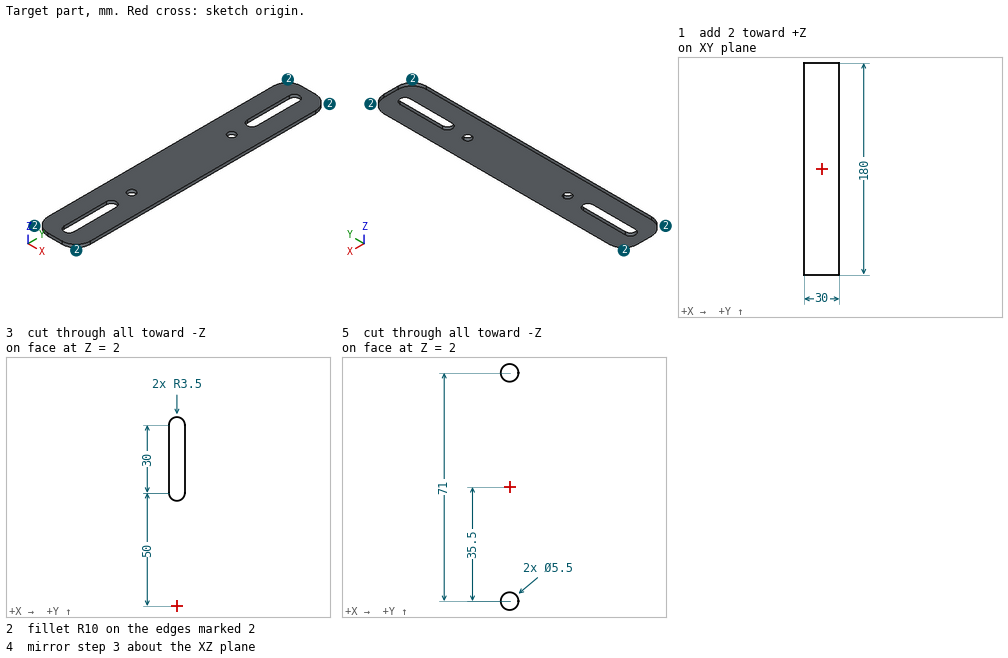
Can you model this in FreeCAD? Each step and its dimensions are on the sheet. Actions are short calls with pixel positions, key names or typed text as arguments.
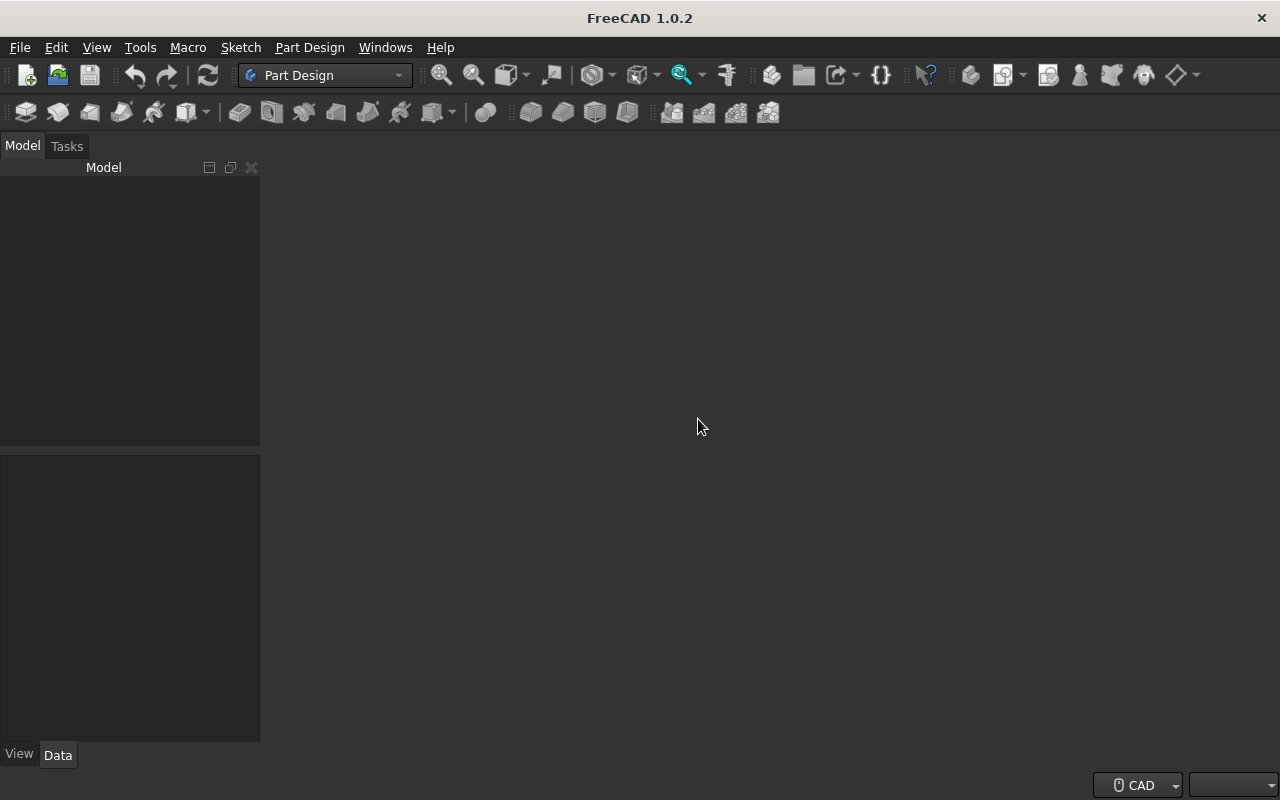
key(ctrl+n)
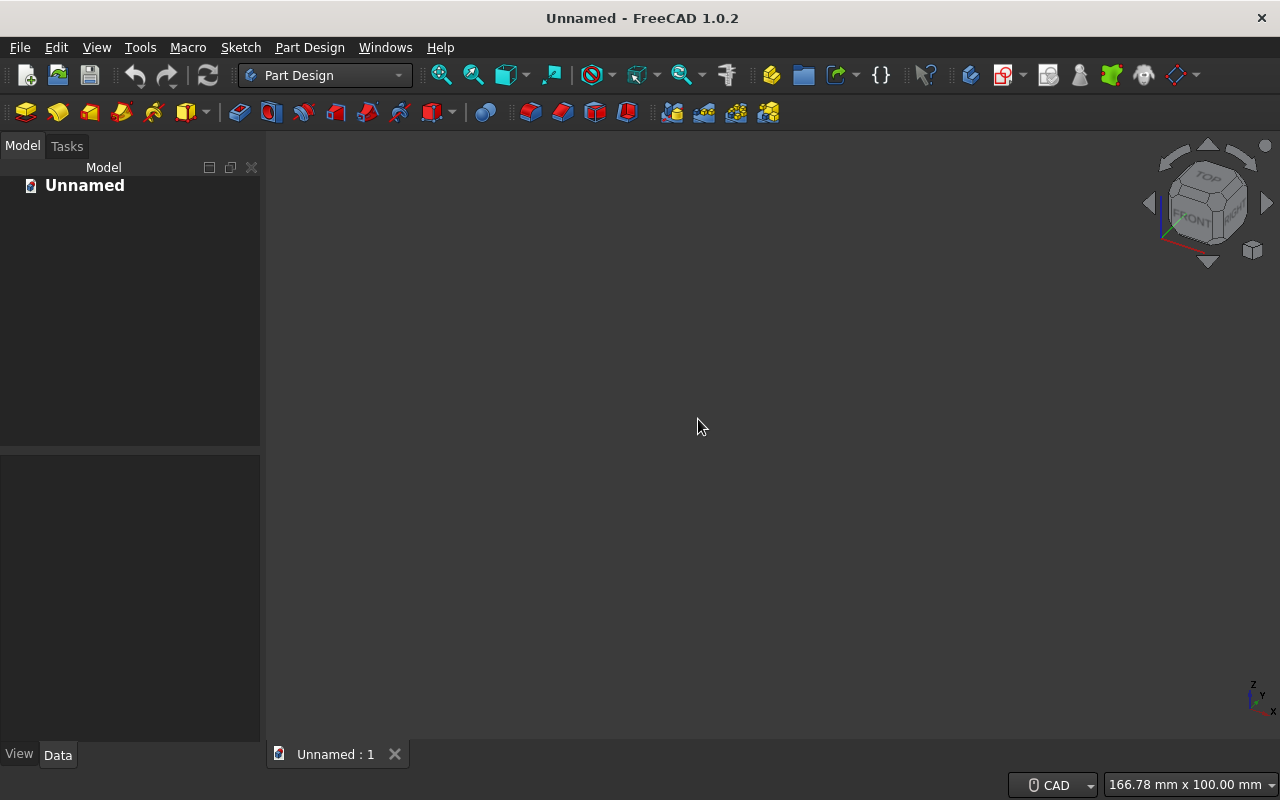
click(1004, 76)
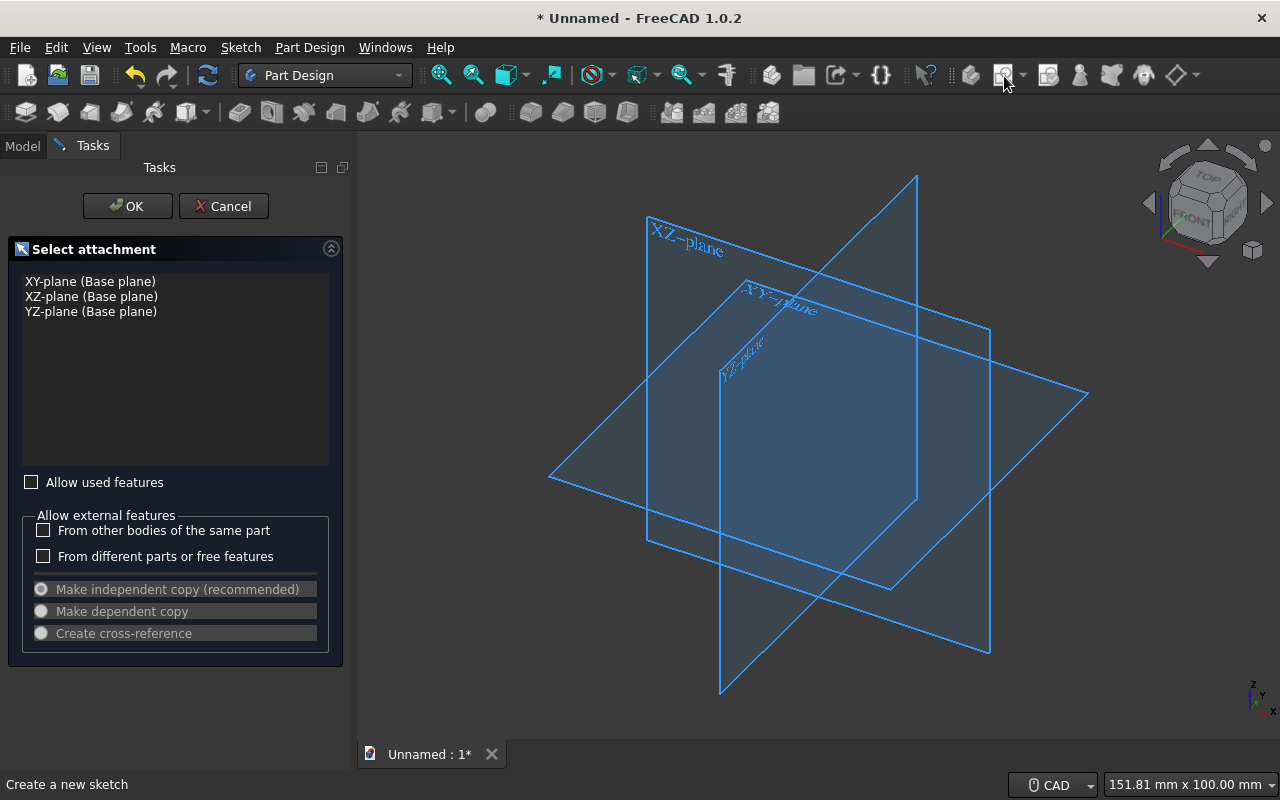
click(82, 282)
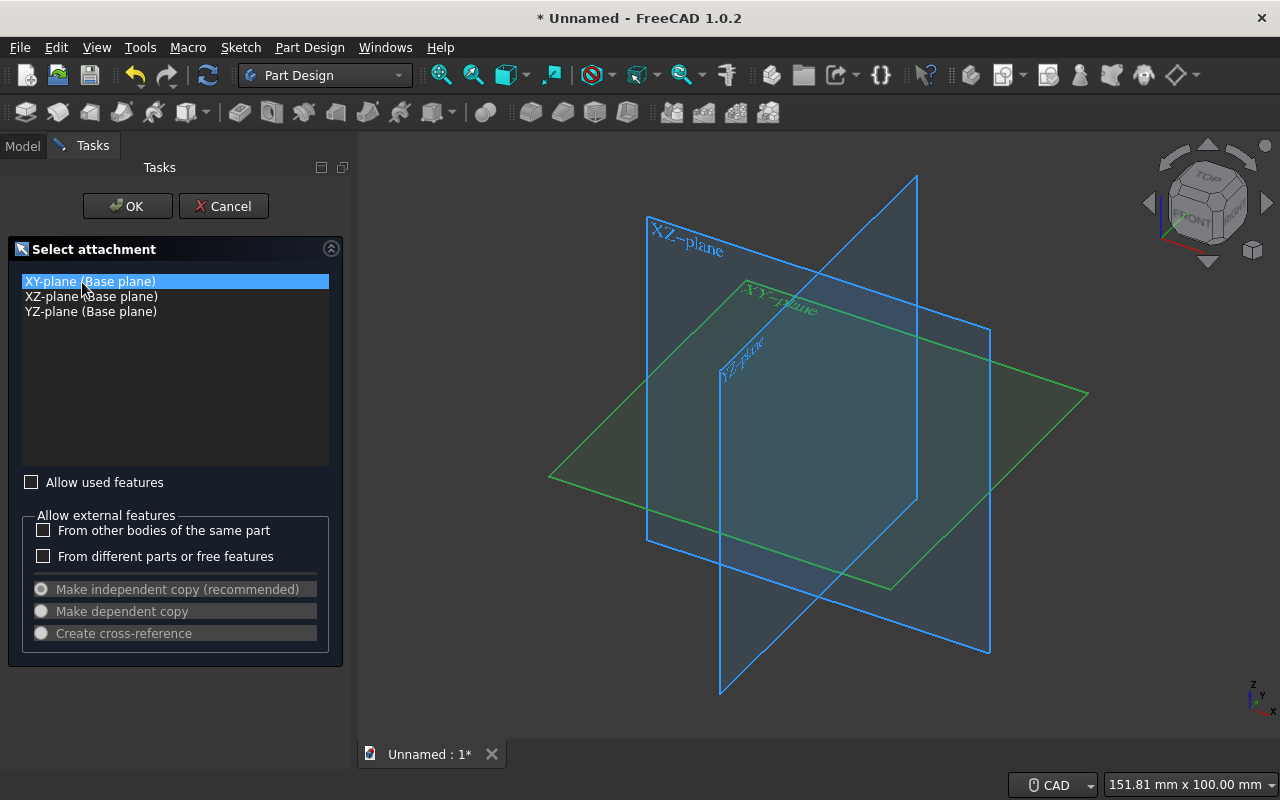
click(128, 206)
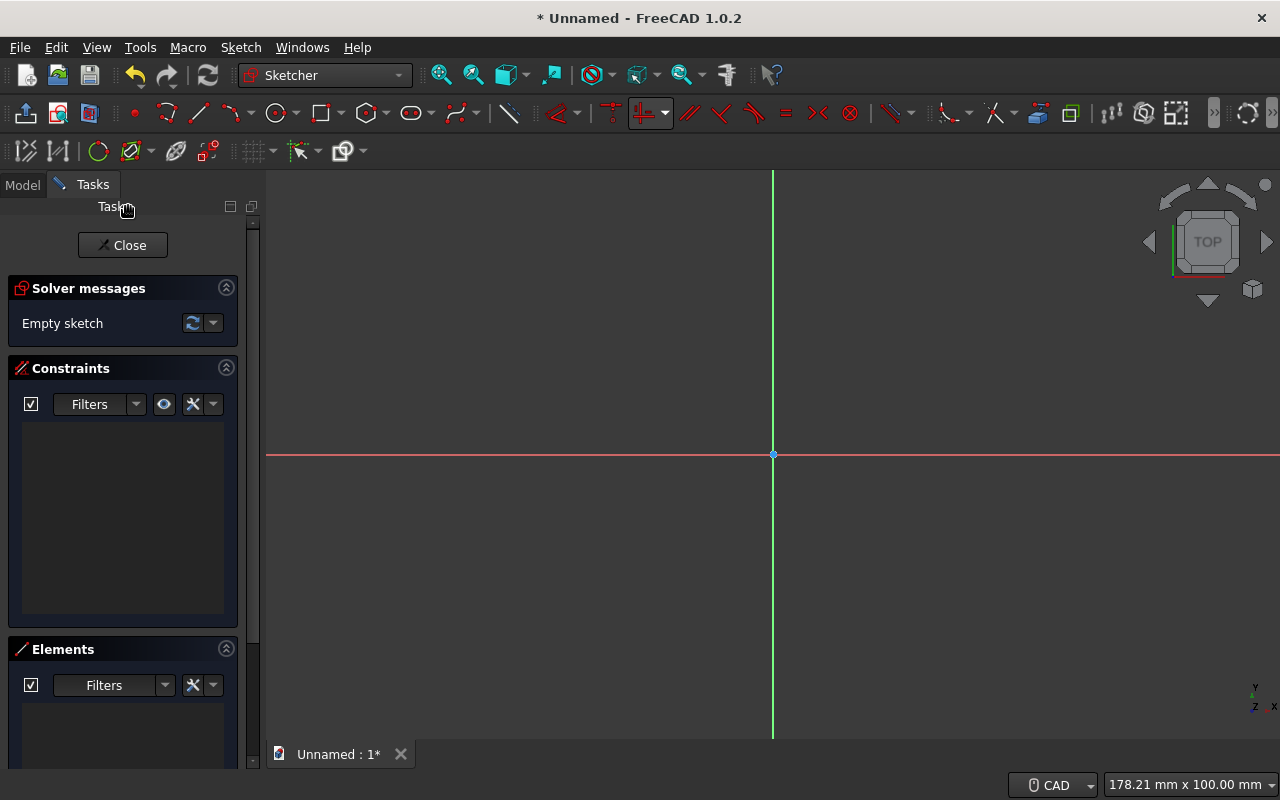
scroll(665, 454, down, 5)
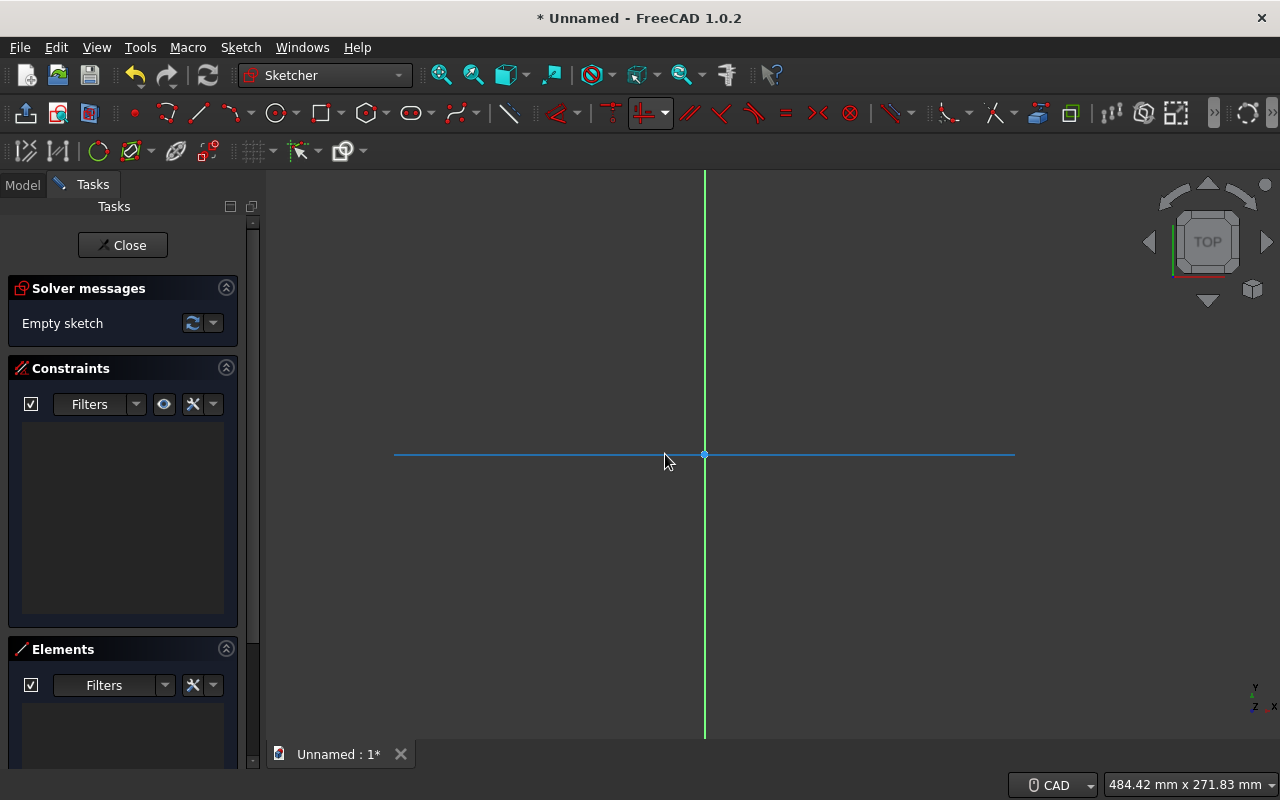
key(g)
key(v)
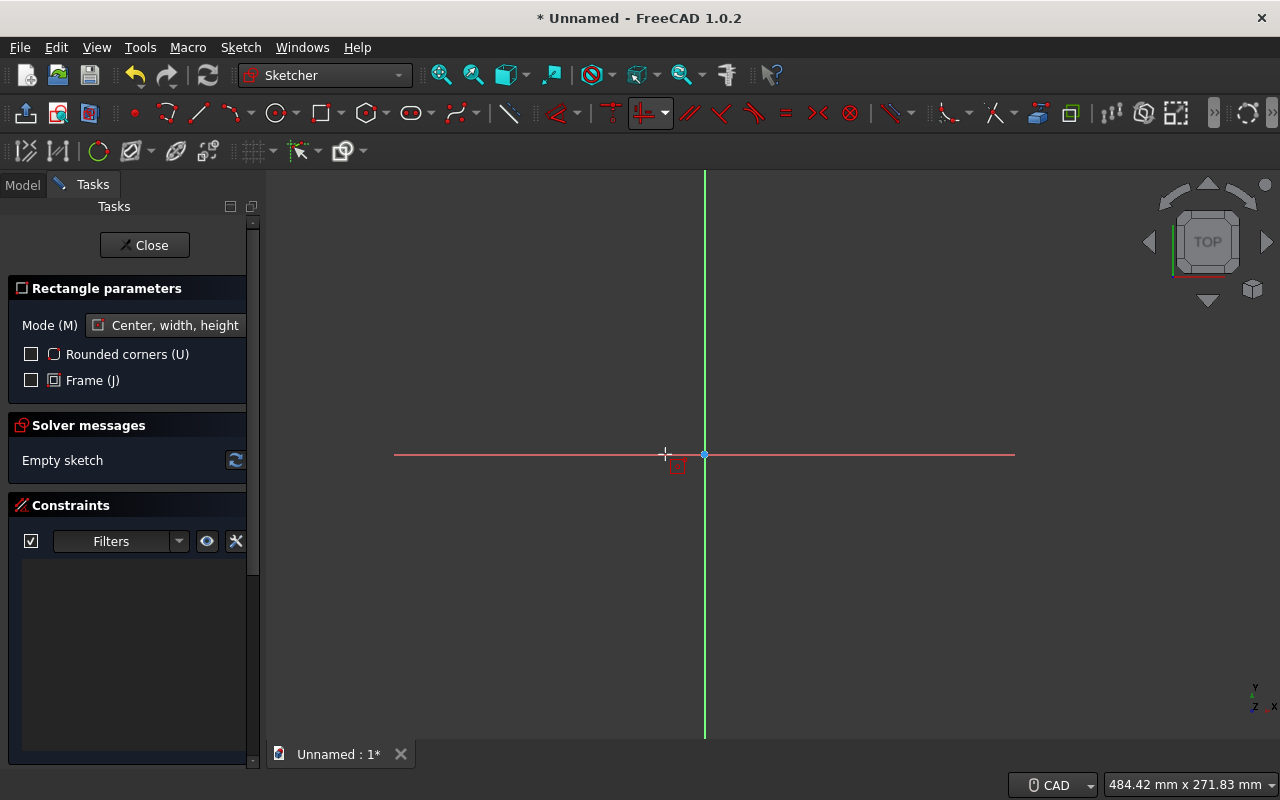
click(705, 454)
click(736, 266)
key(Escape)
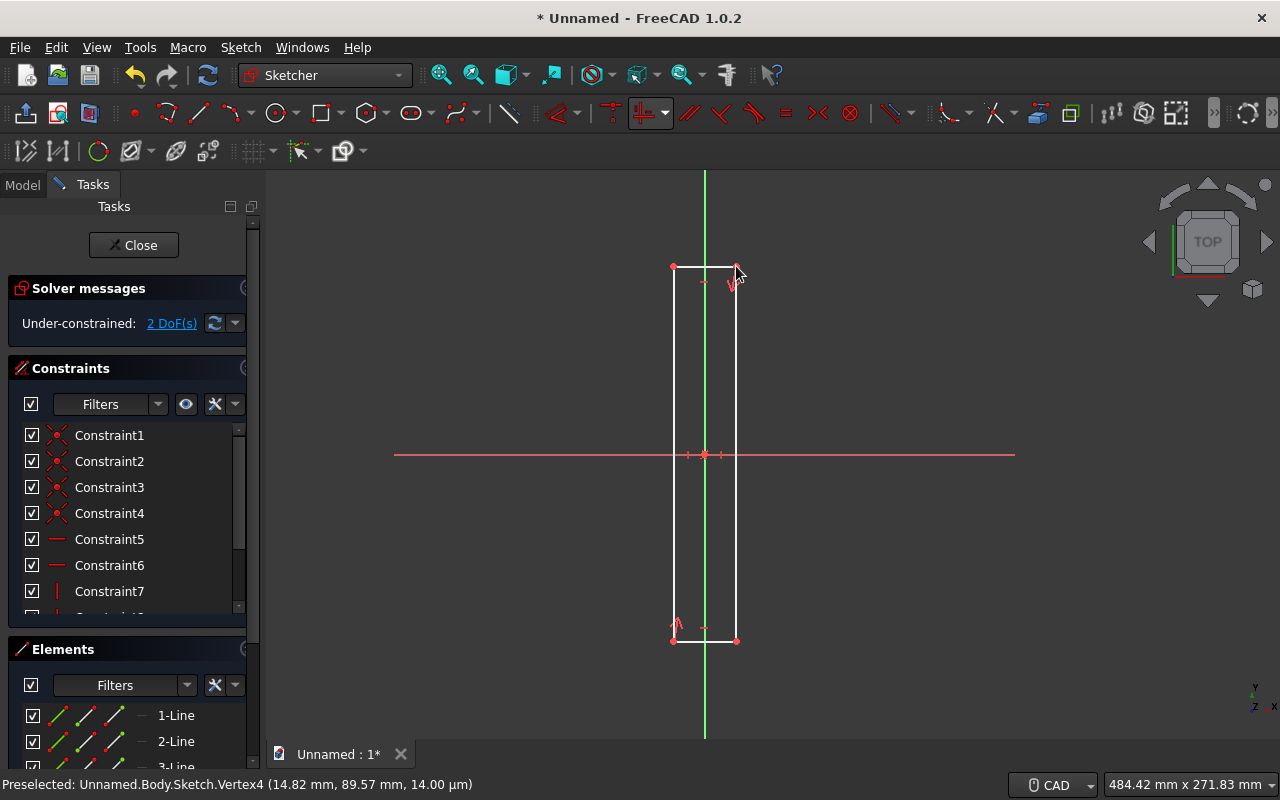
key(d)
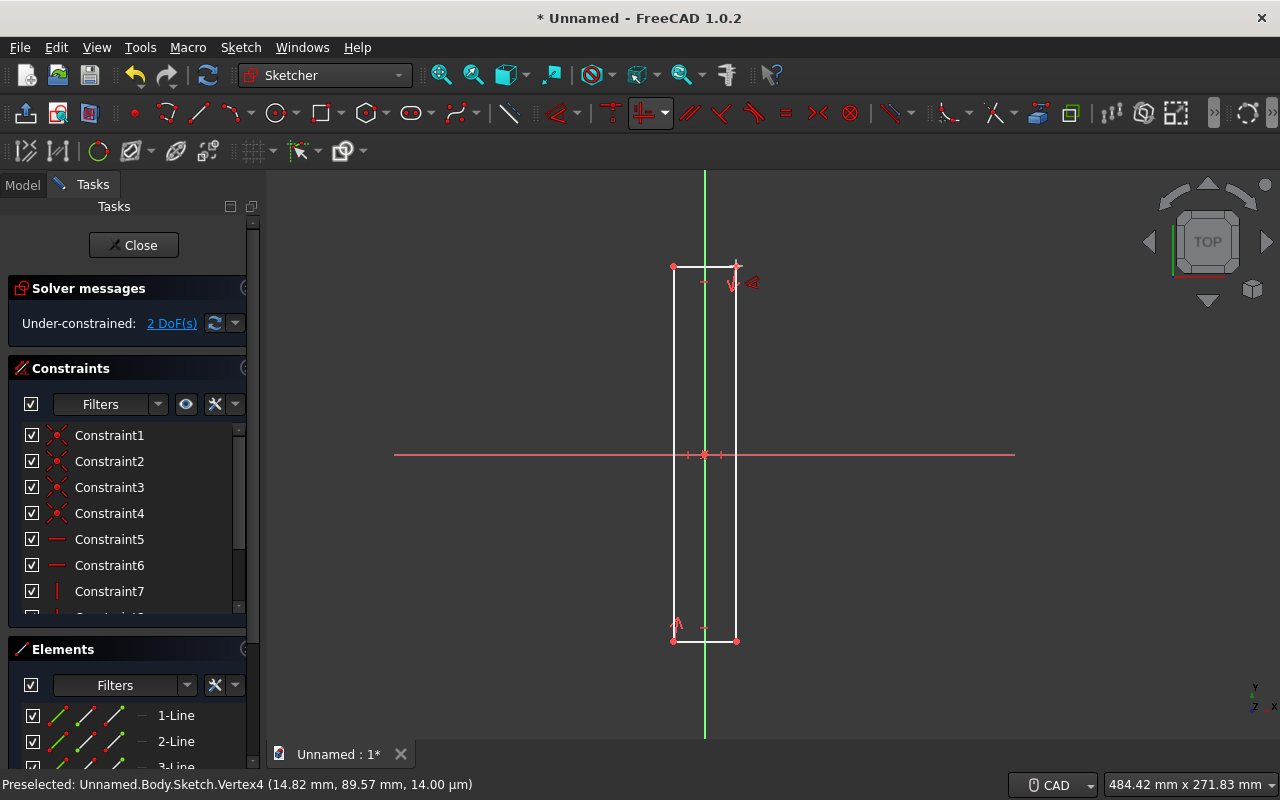
click(693, 642)
click(691, 676)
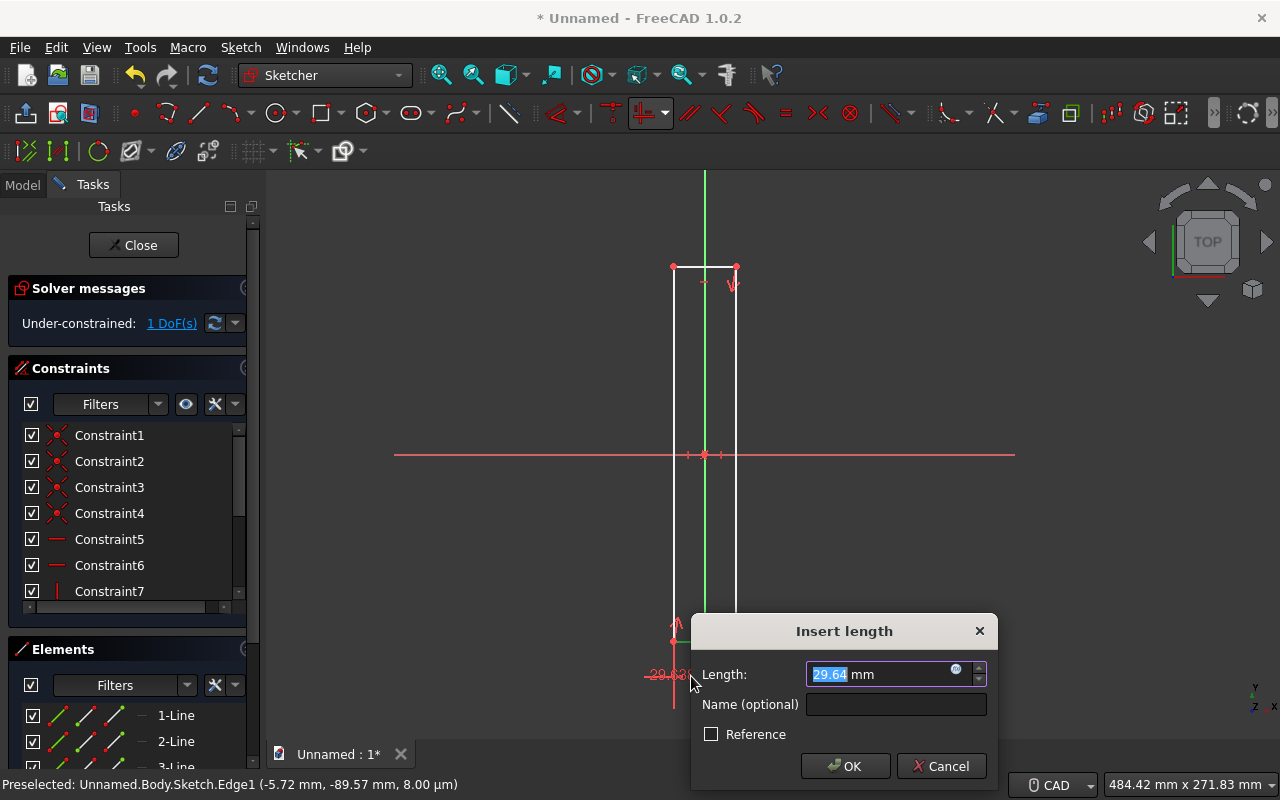
text(30)
key(Return)